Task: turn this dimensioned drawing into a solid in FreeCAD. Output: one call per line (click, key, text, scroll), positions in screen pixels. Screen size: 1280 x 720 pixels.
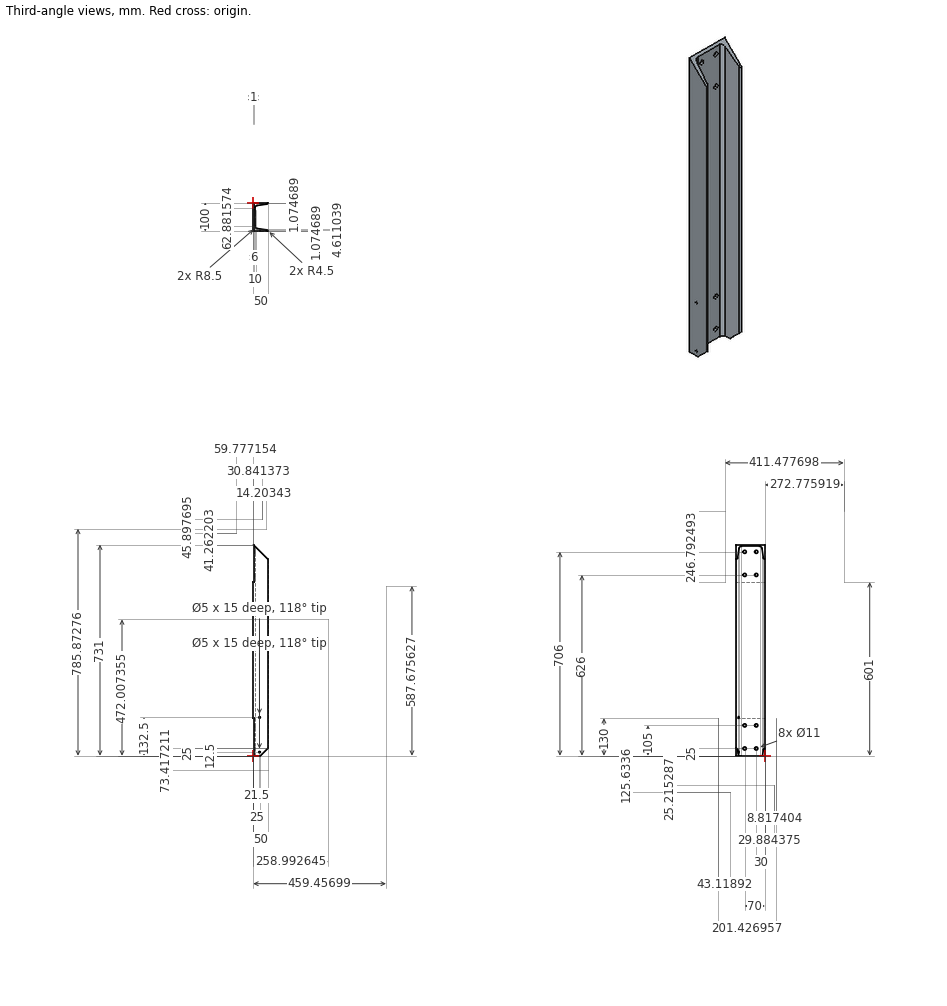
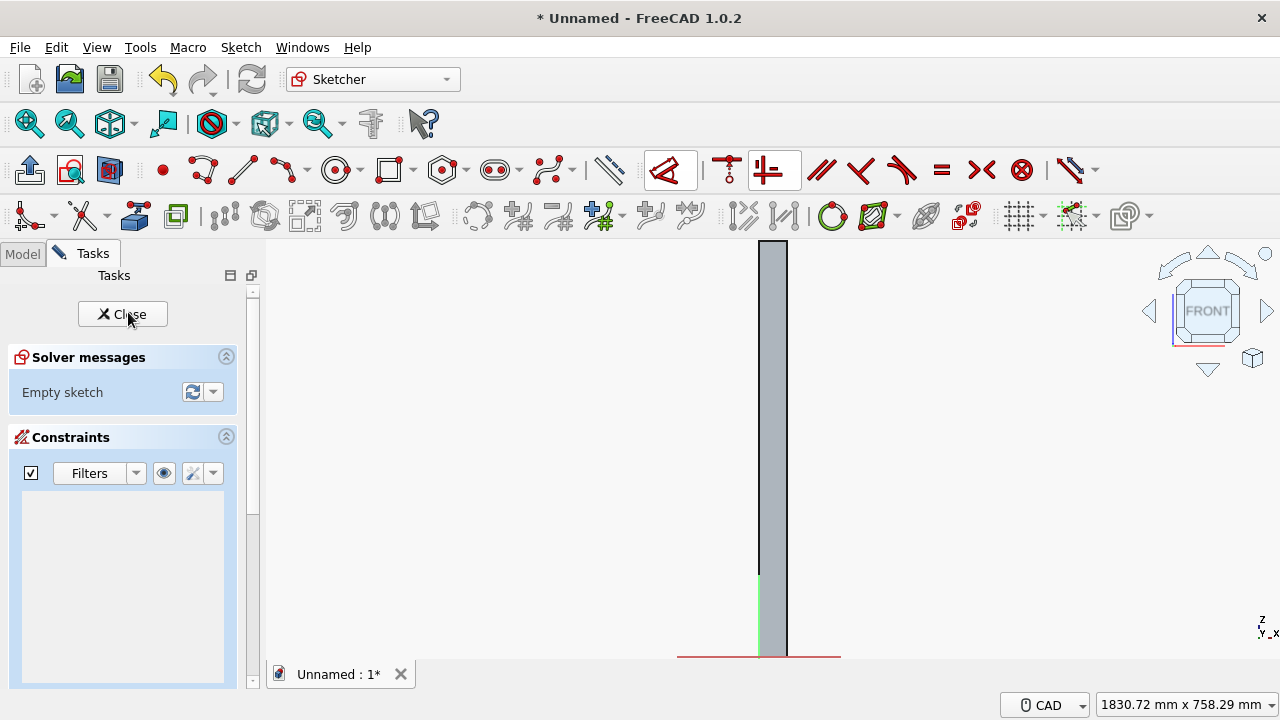
scroll(503, 456, down, 3)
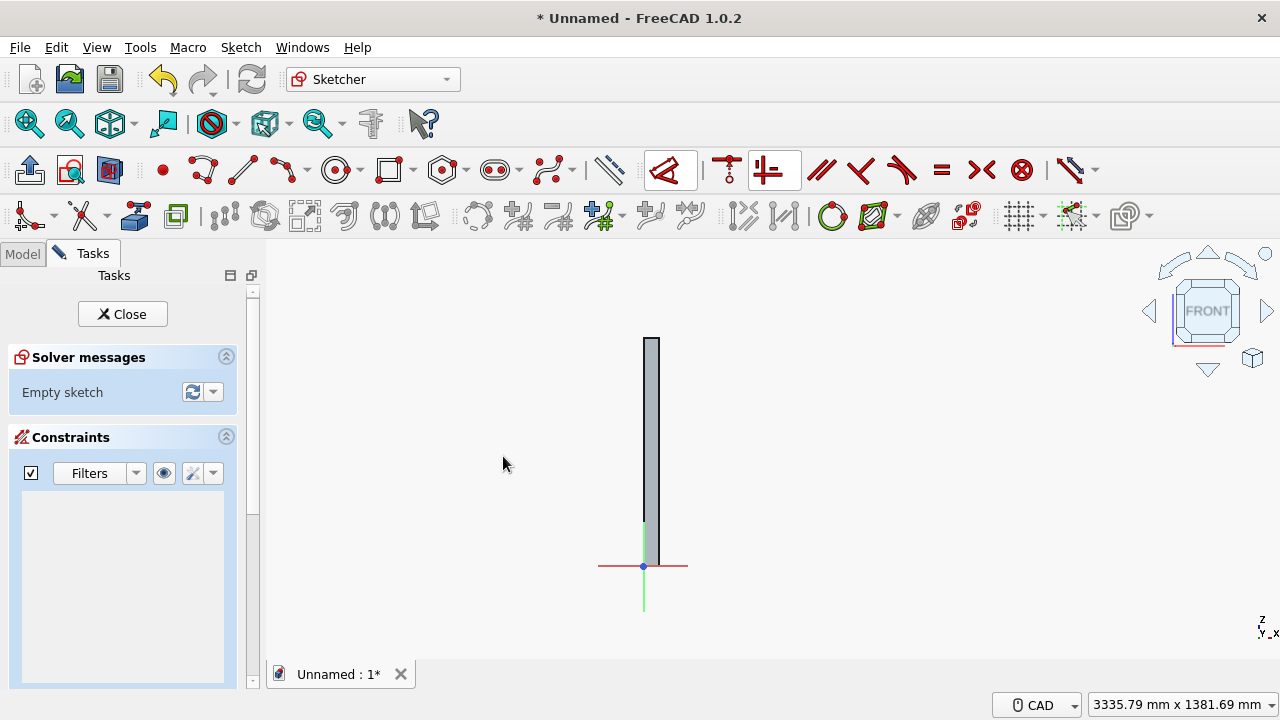
key(g)
key(m)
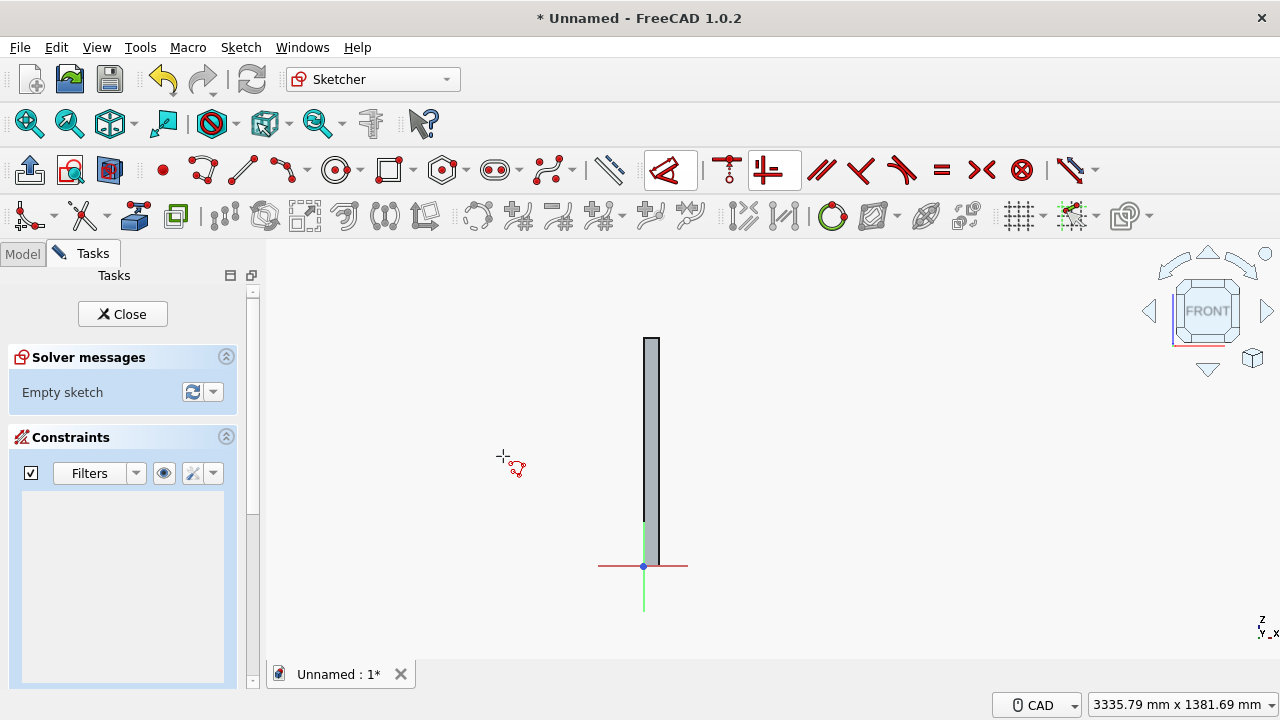
click(722, 423)
click(644, 344)
click(626, 332)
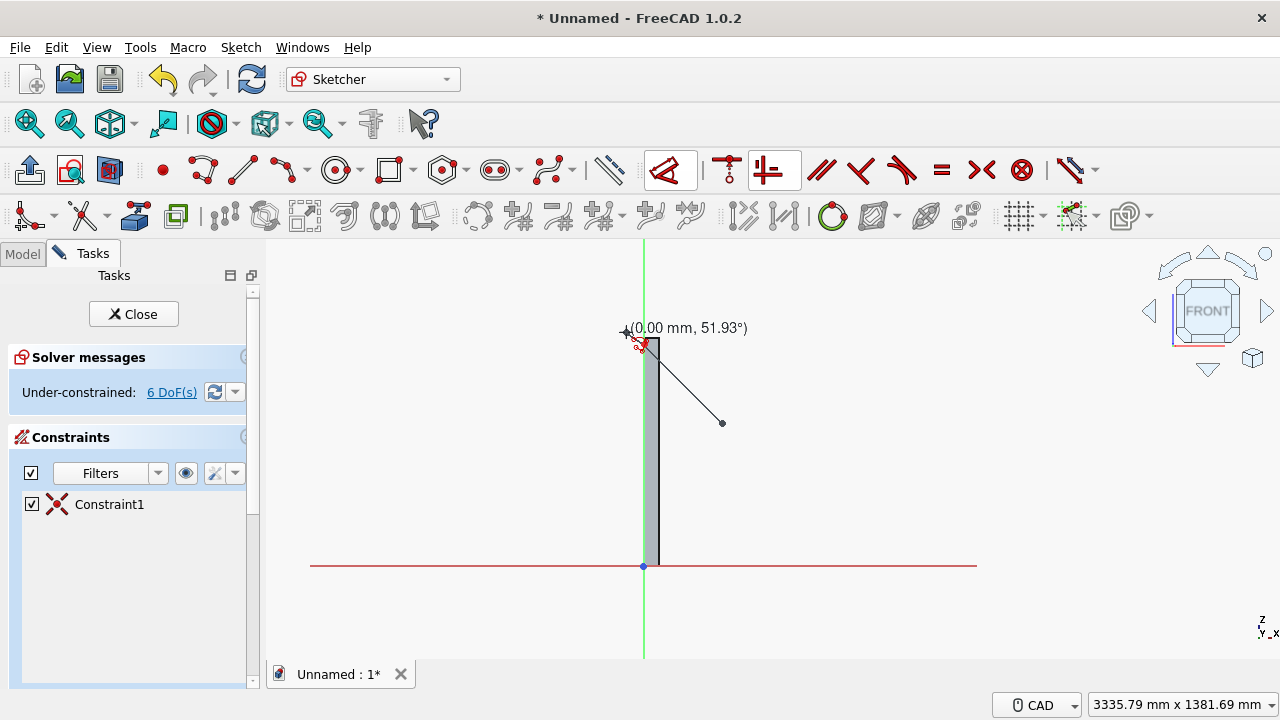
scroll(653, 318, up, 3)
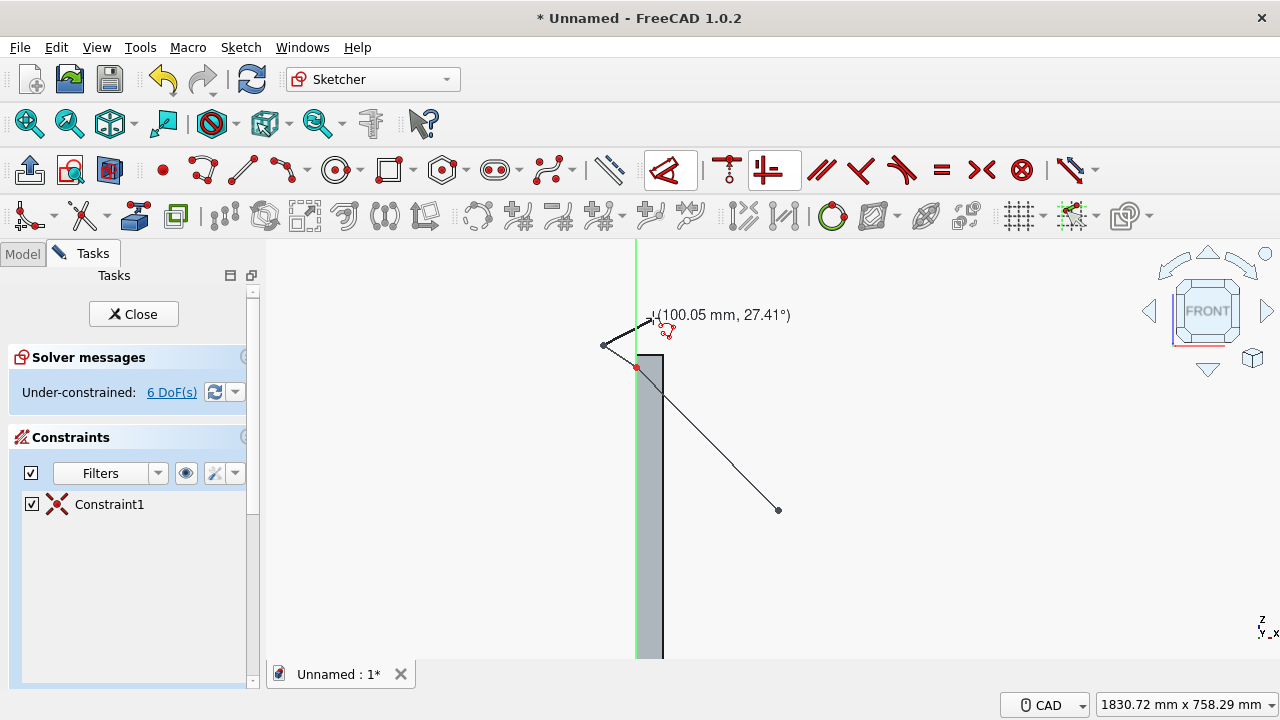
click(653, 317)
click(661, 335)
click(890, 445)
click(778, 511)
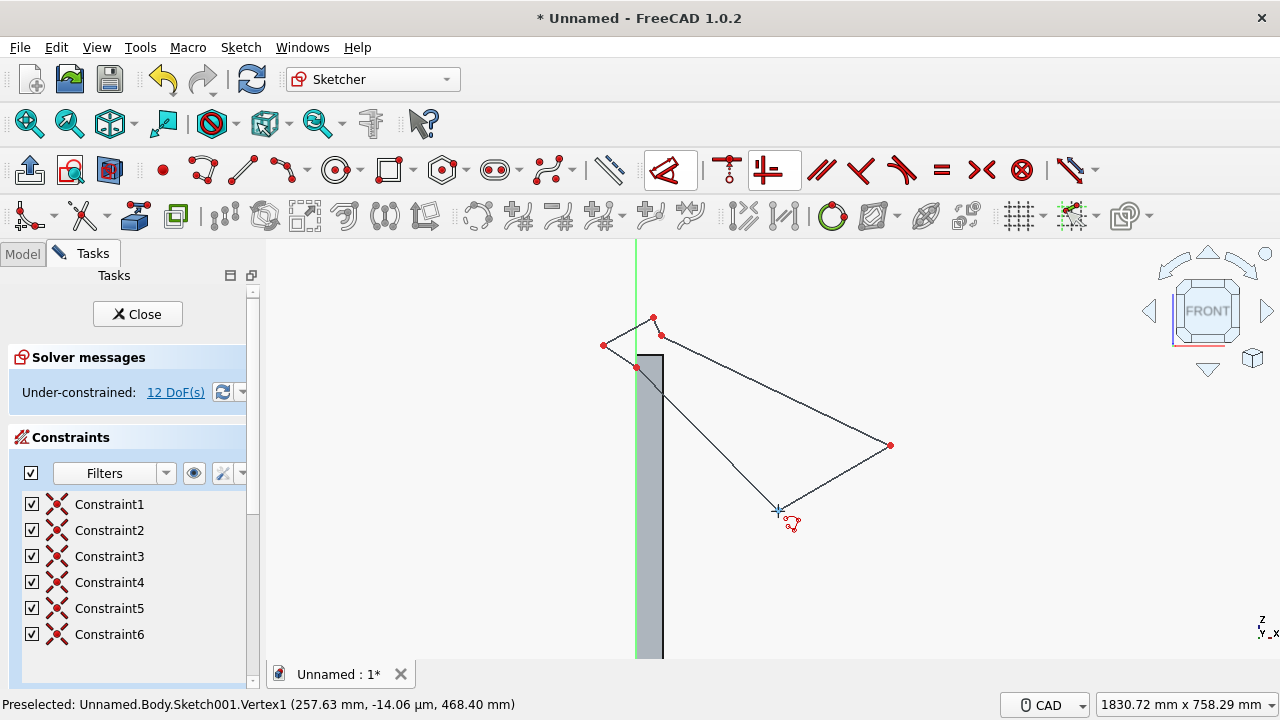
scroll(654, 317, down, 3)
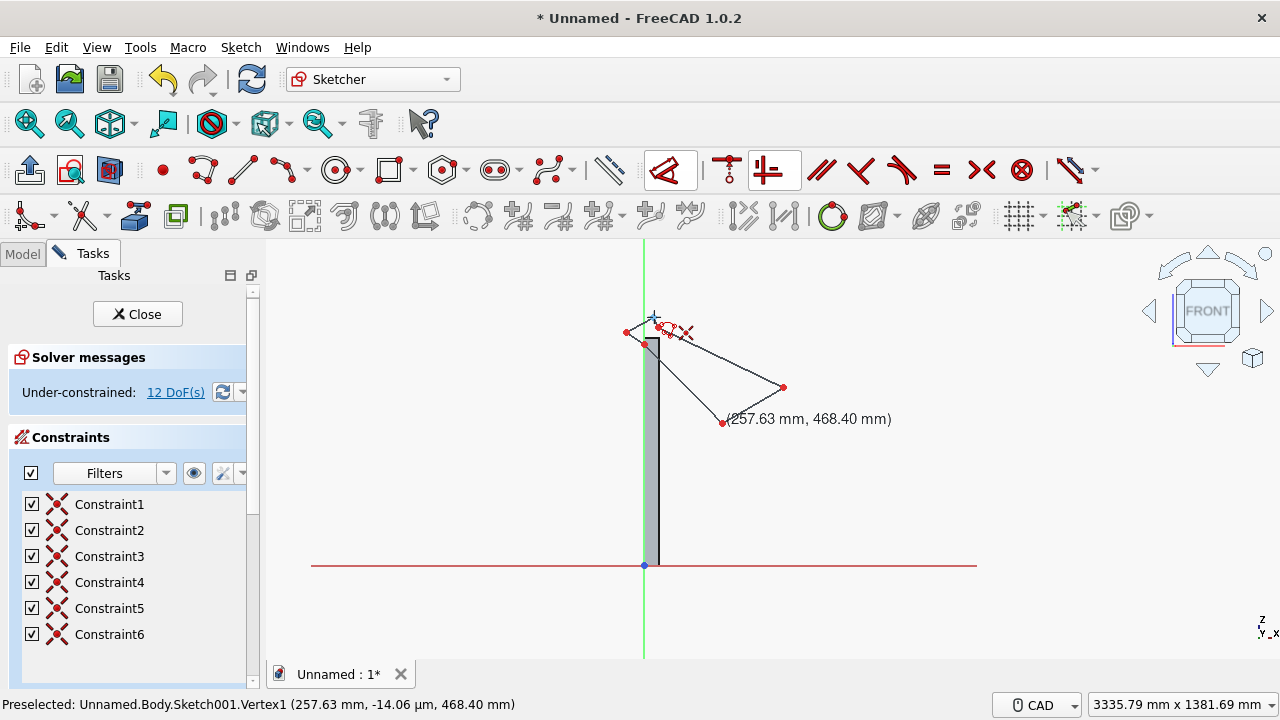
scroll(652, 566, up, 4)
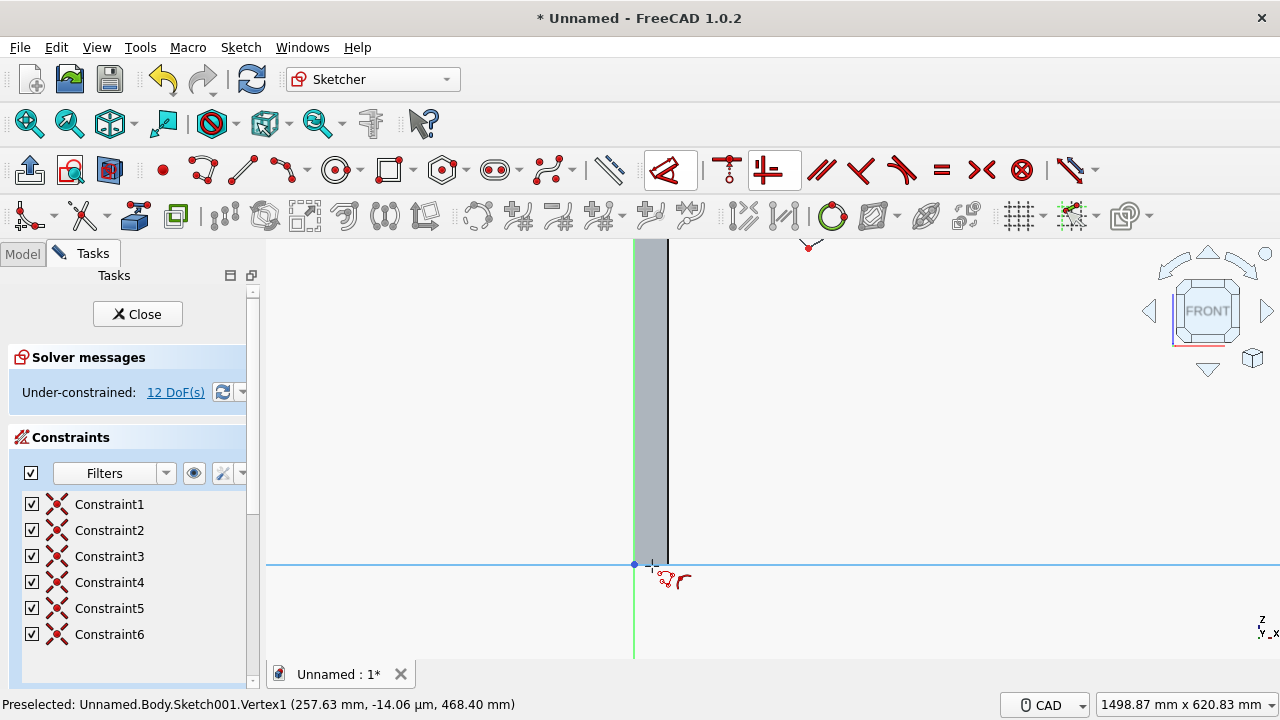
click(651, 565)
click(668, 548)
click(668, 598)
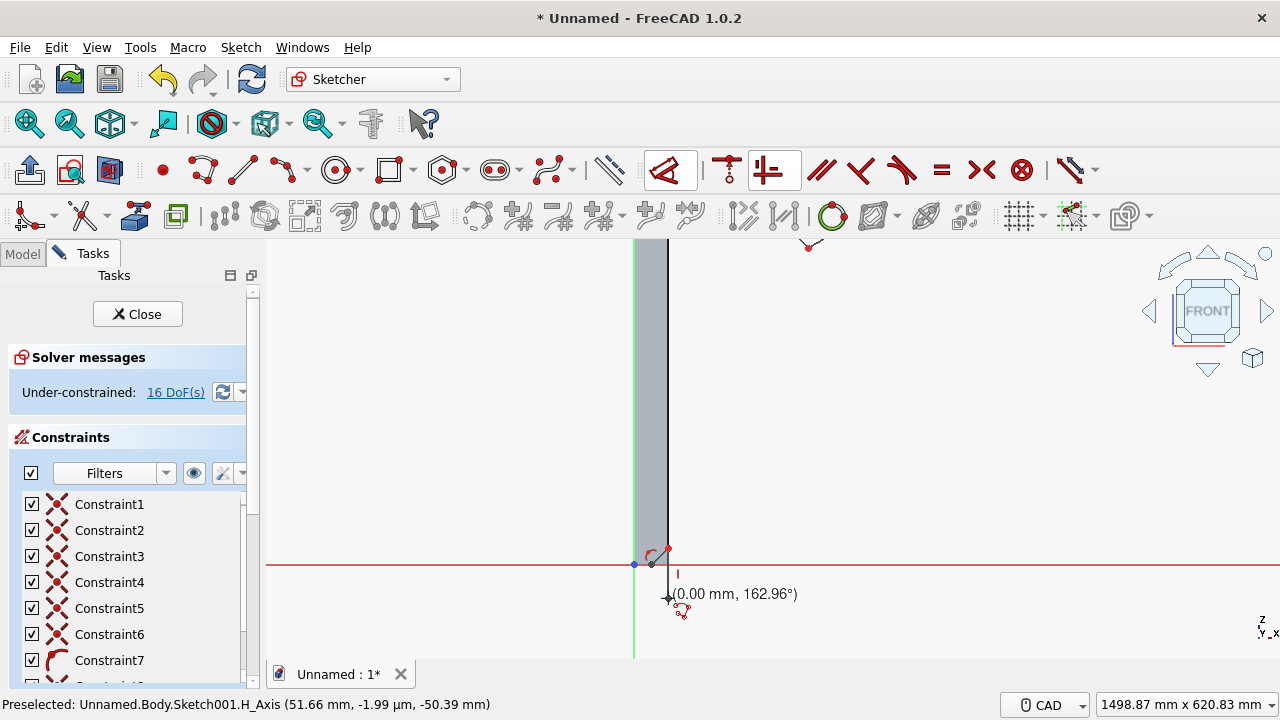
scroll(651, 565, up, 2)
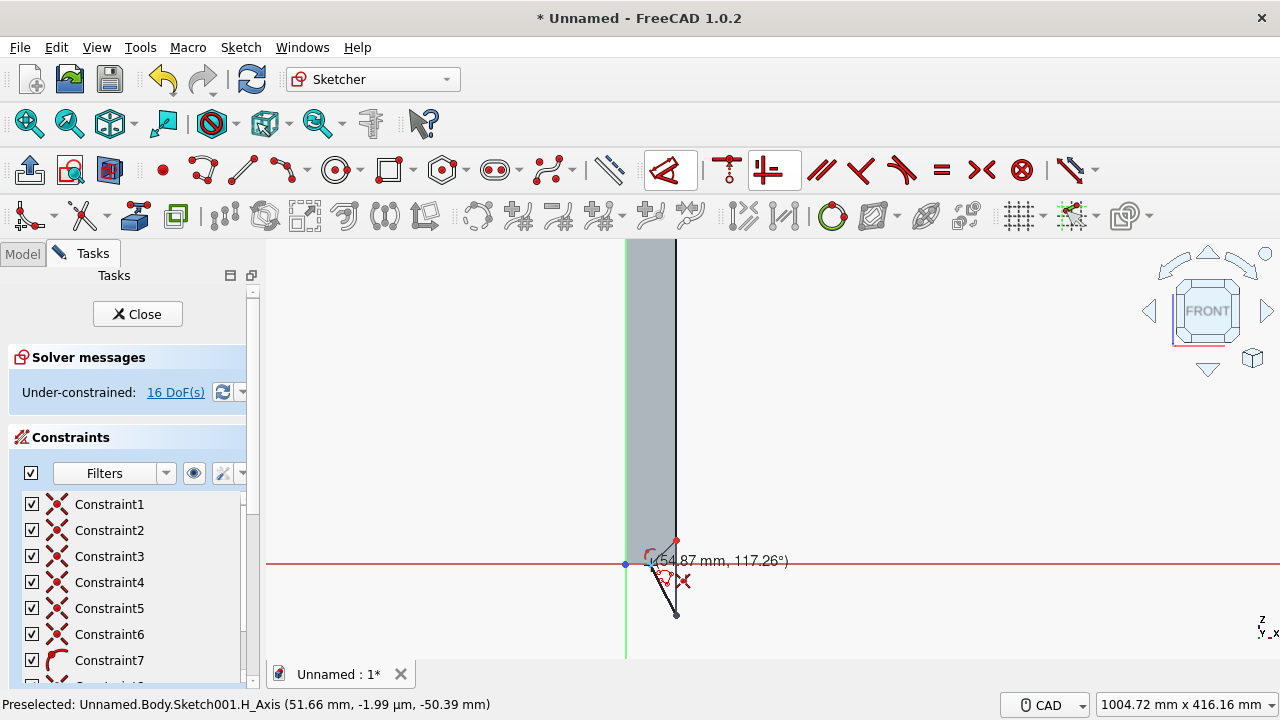
click(651, 564)
key(Escape)
key(Escape)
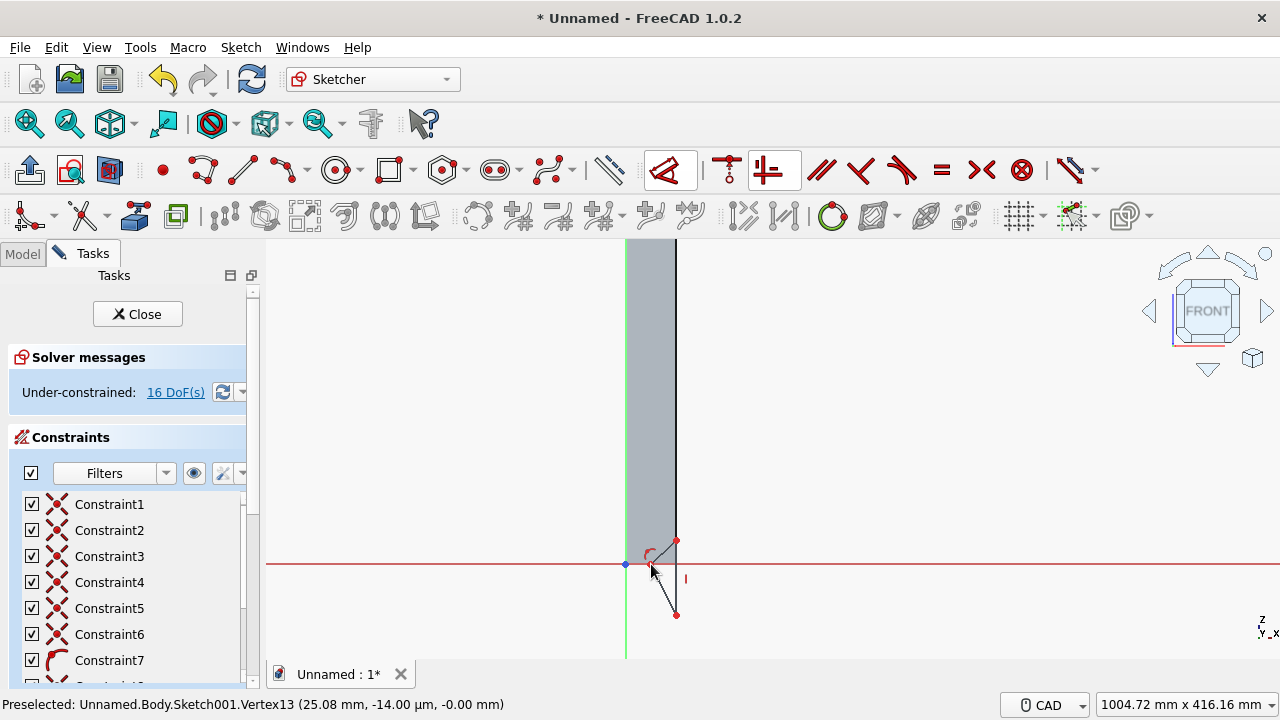
scroll(652, 567, down, 6)